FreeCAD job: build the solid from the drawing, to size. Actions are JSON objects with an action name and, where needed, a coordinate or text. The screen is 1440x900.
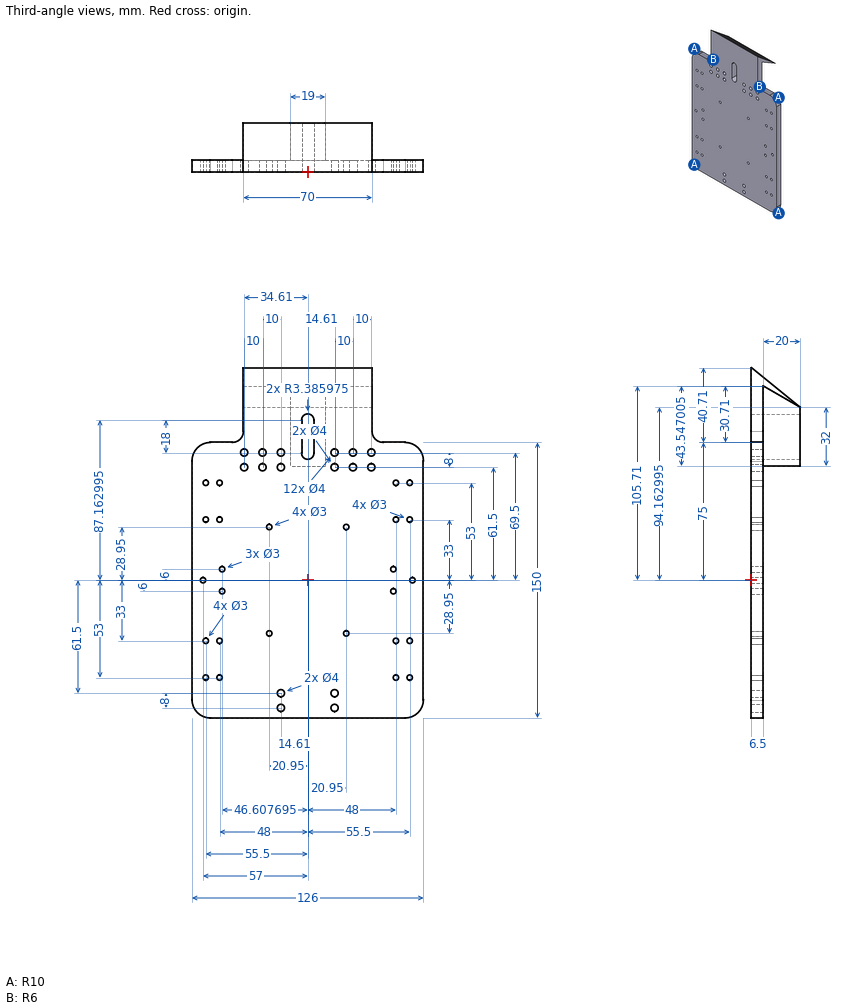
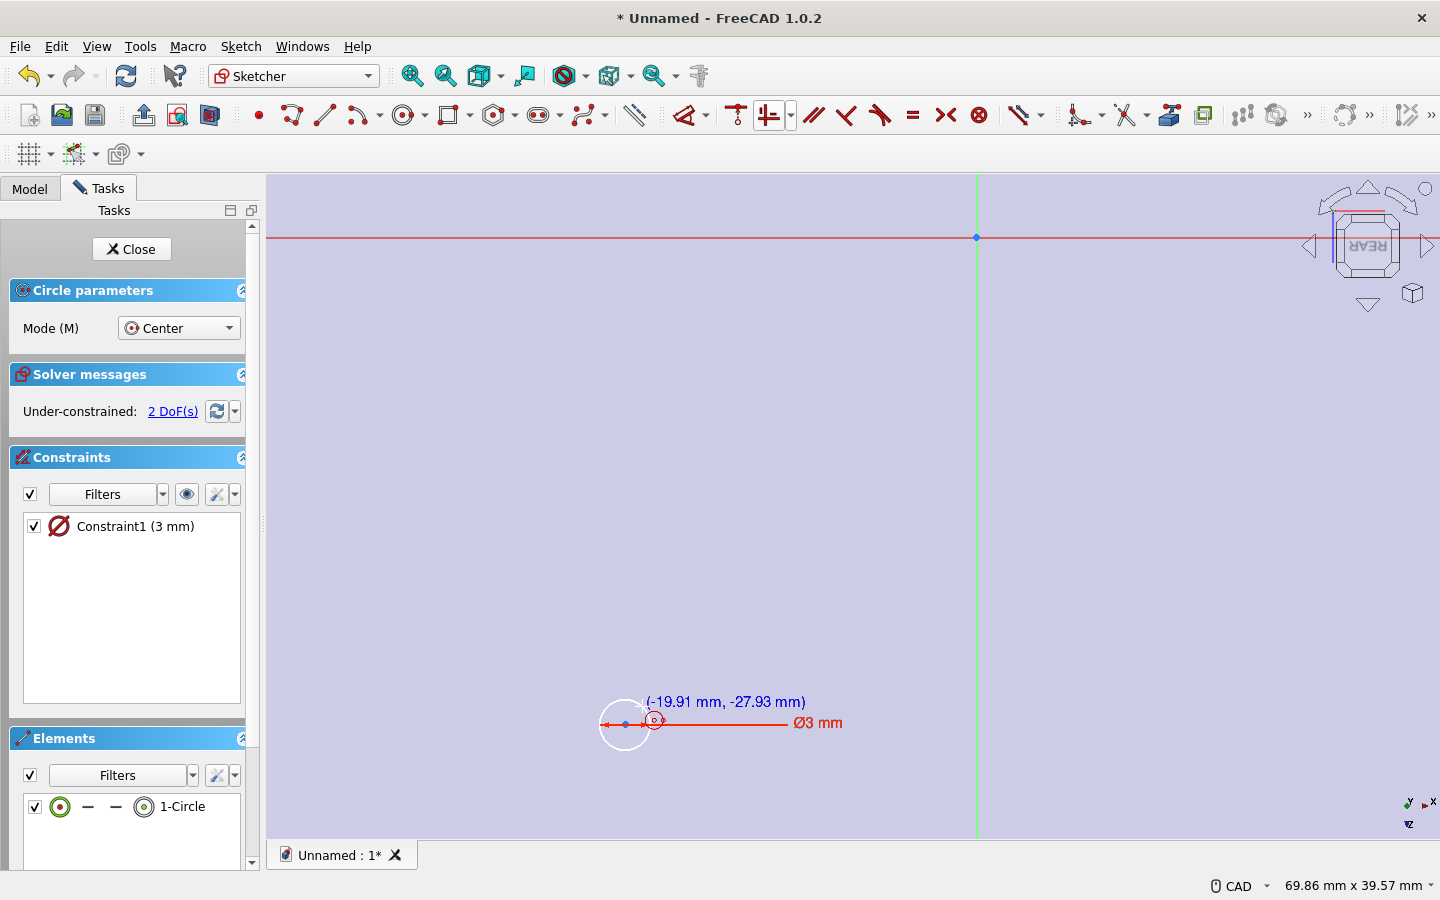
{"action": "scroll", "coordinate": [628, 726], "scroll_direction": "down", "scroll_amount": 4}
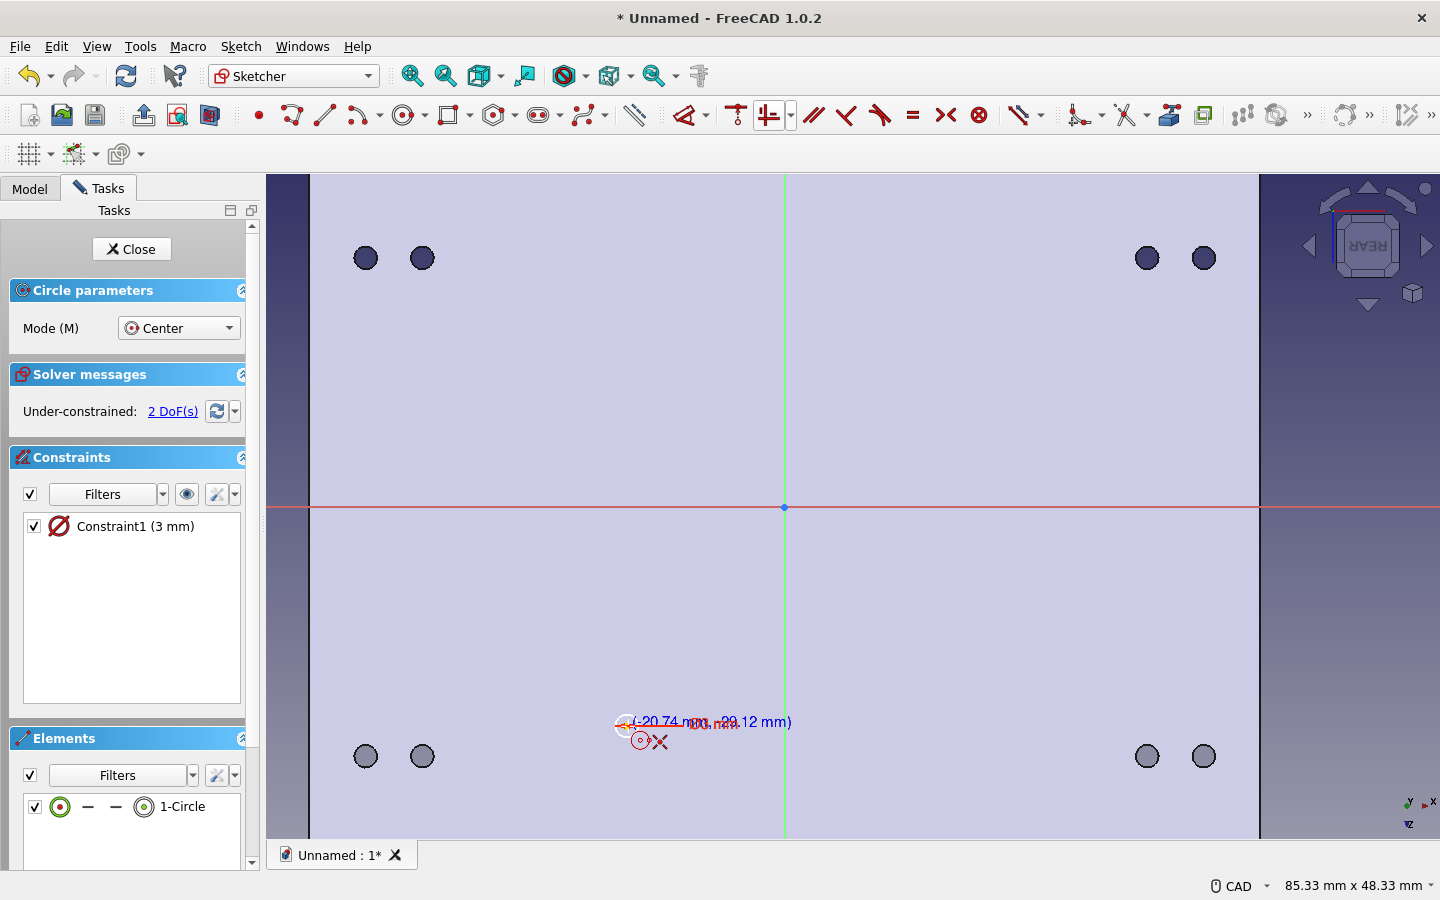
{"action": "scroll", "coordinate": [943, 726], "scroll_direction": "up", "scroll_amount": 4}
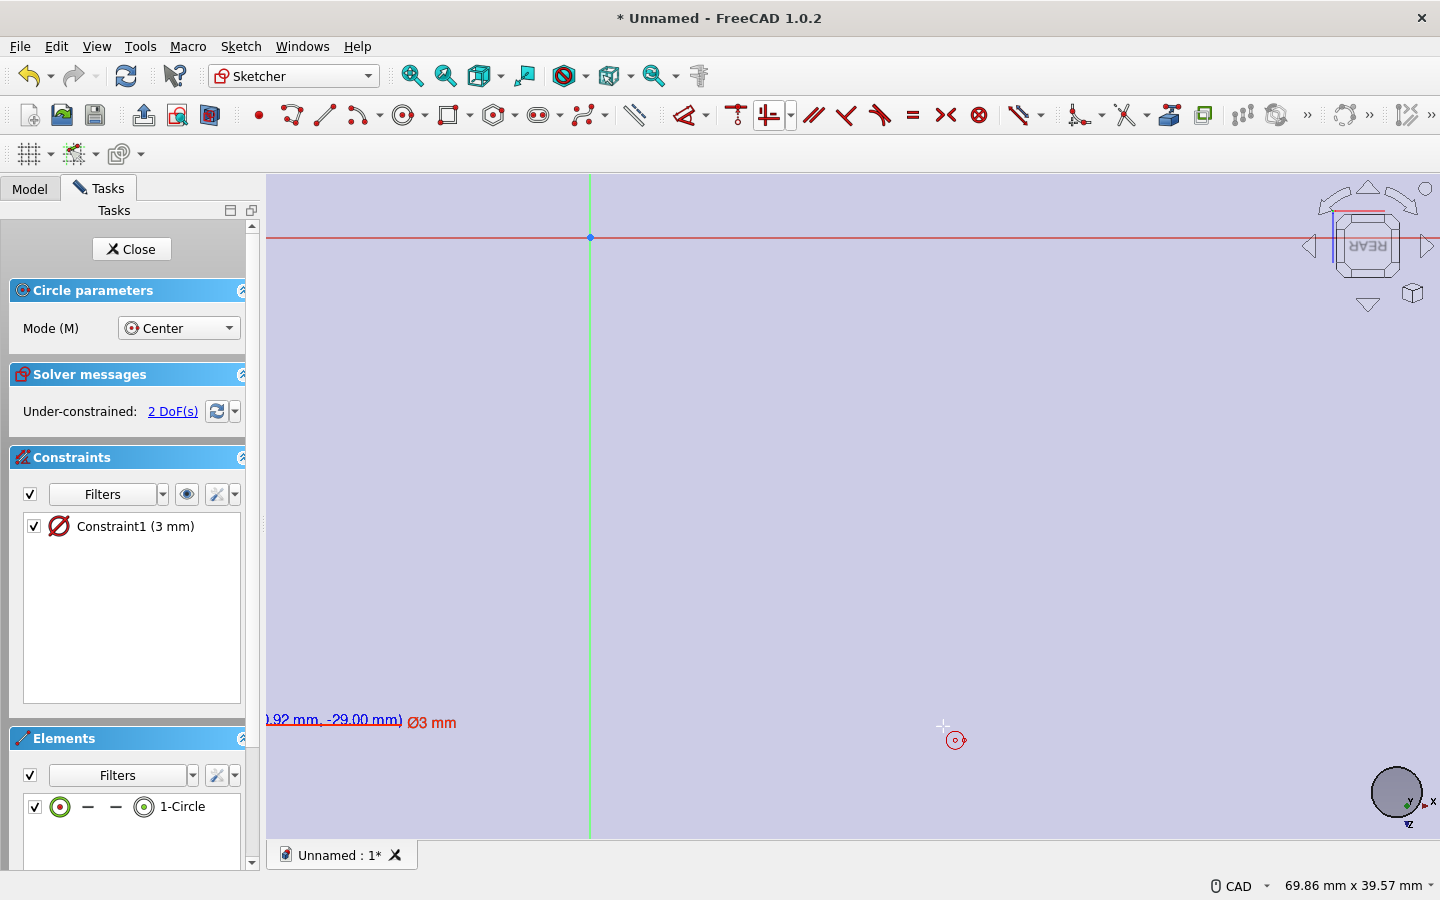
{"action": "left_click", "coordinate": [942, 724]}
{"action": "mouse_move", "coordinate": [960, 706]}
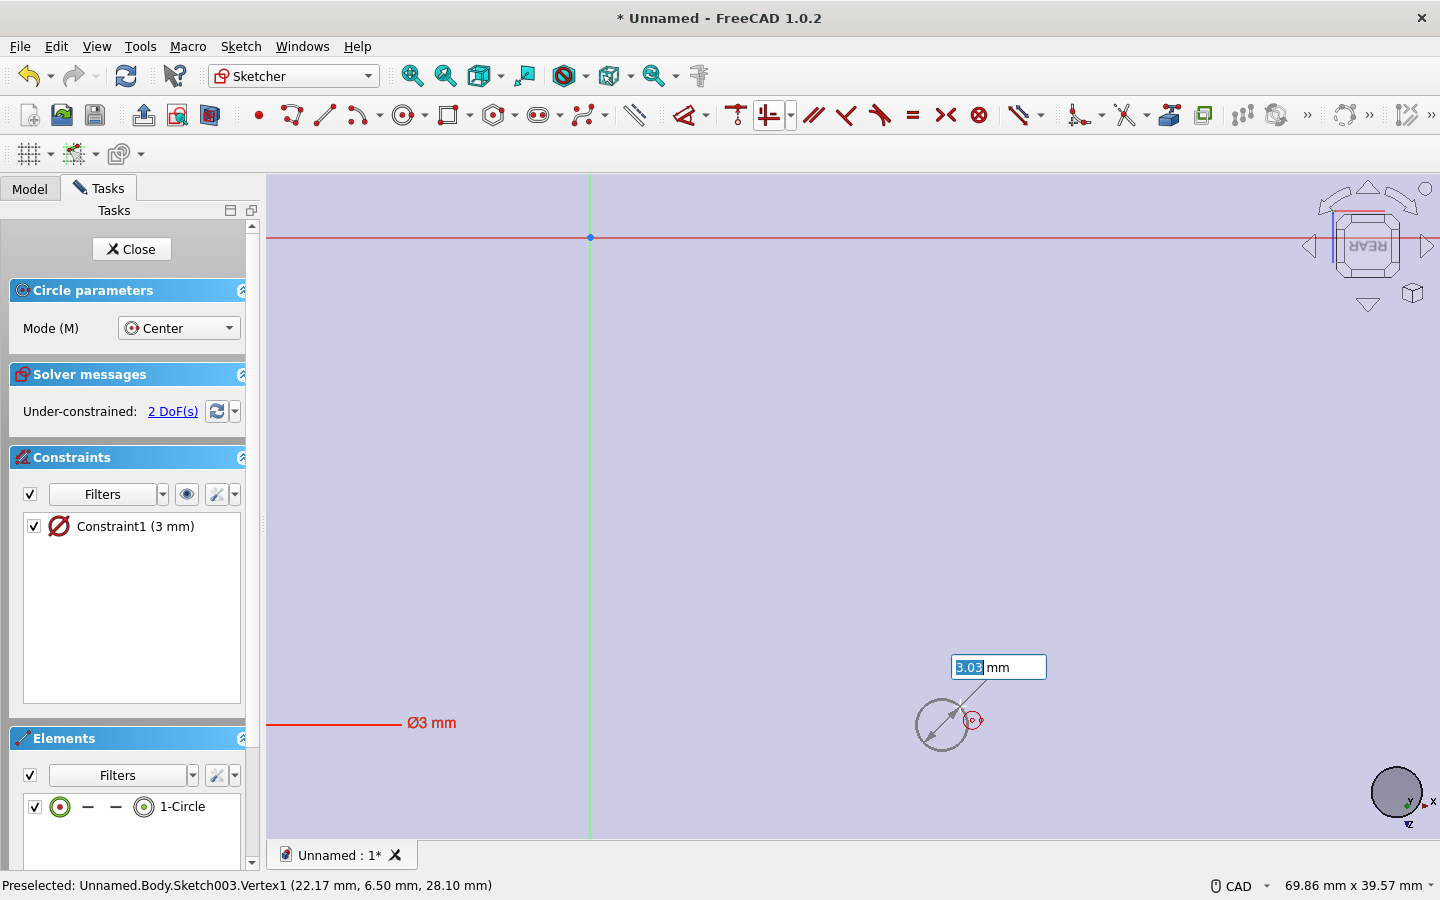
{"action": "type", "text": "3"}
{"action": "key", "text": "Return"}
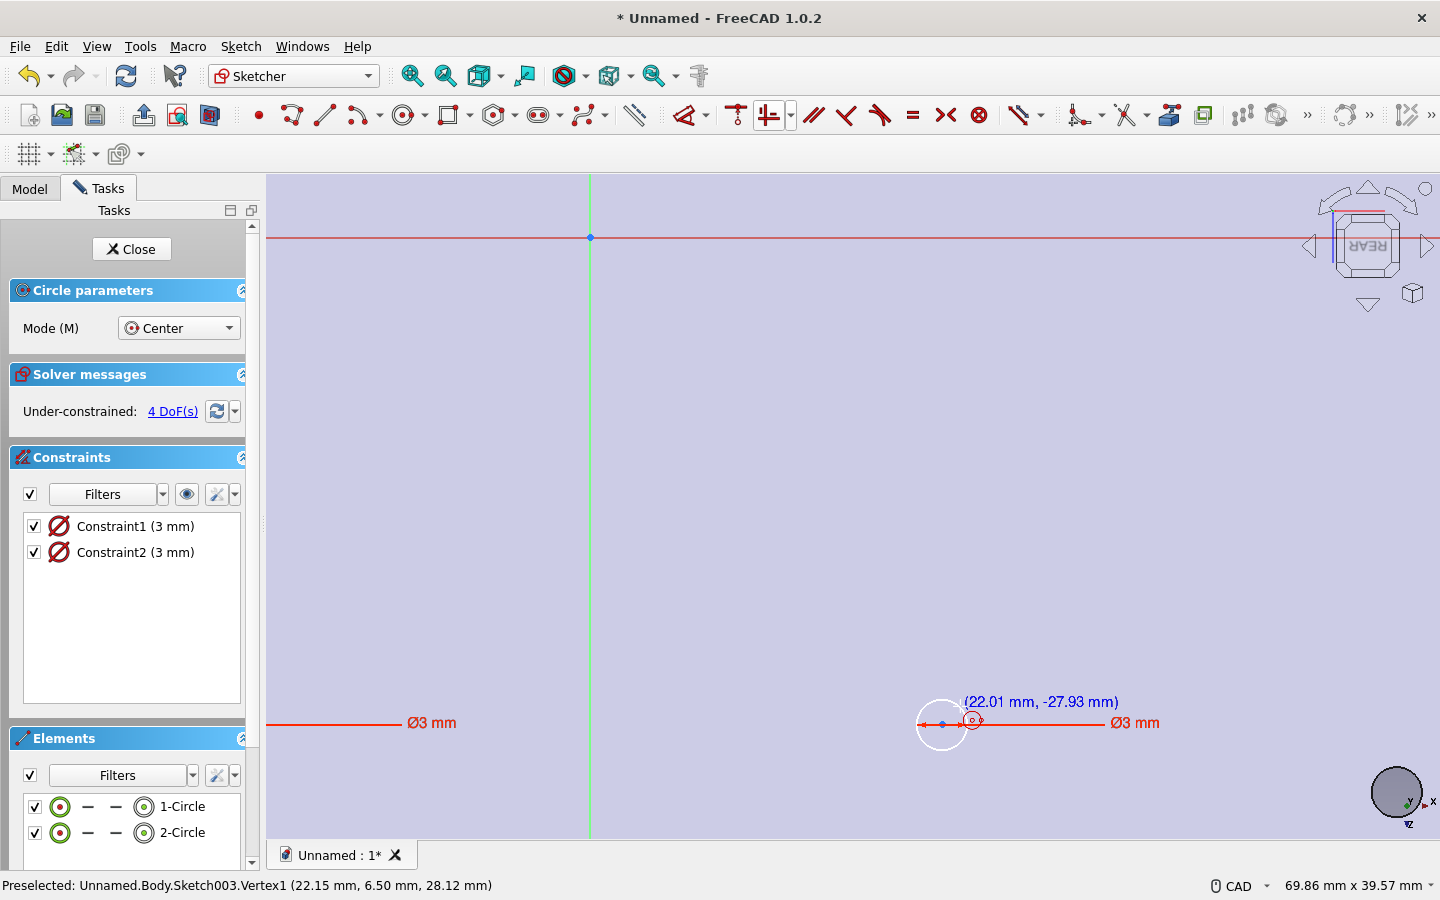
{"action": "scroll", "coordinate": [943, 726], "scroll_direction": "down", "scroll_amount": 4}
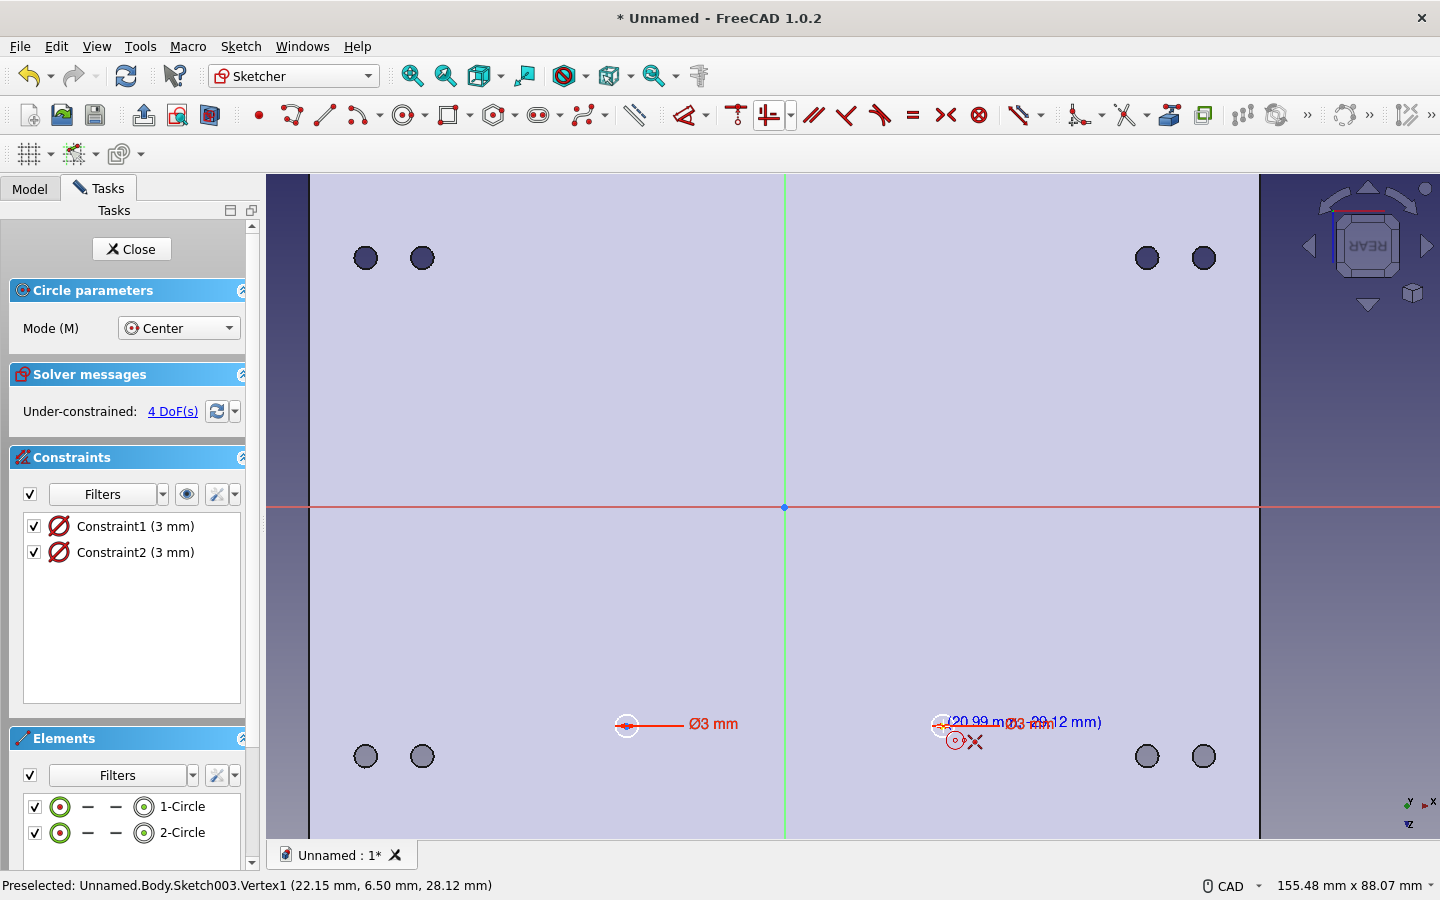
{"action": "scroll", "coordinate": [943, 288], "scroll_direction": "up", "scroll_amount": 4}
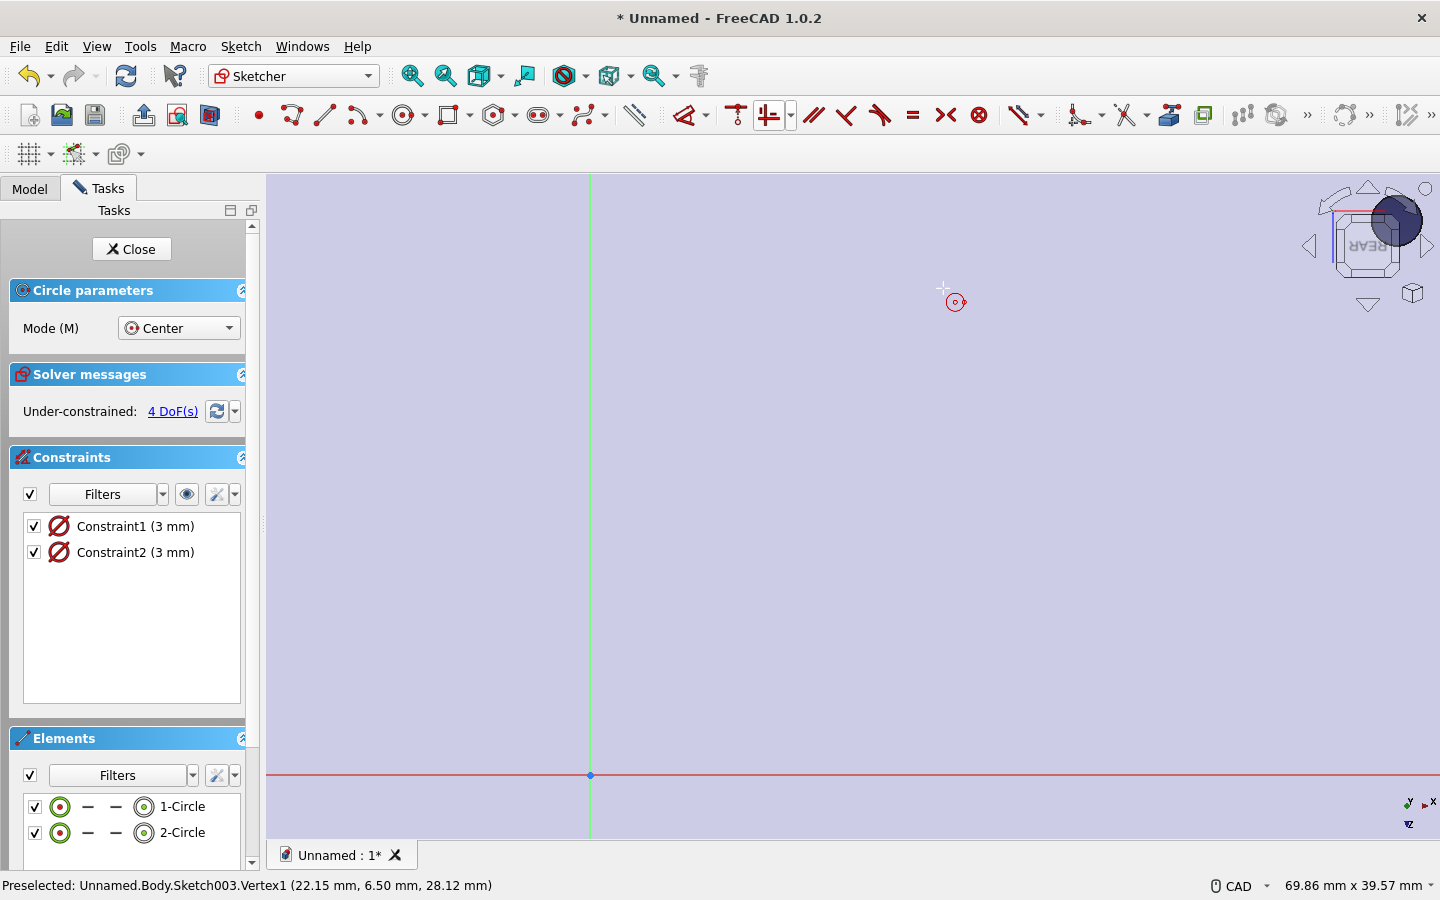
{"action": "left_click", "coordinate": [942, 289]}
{"action": "mouse_move", "coordinate": [960, 271]}